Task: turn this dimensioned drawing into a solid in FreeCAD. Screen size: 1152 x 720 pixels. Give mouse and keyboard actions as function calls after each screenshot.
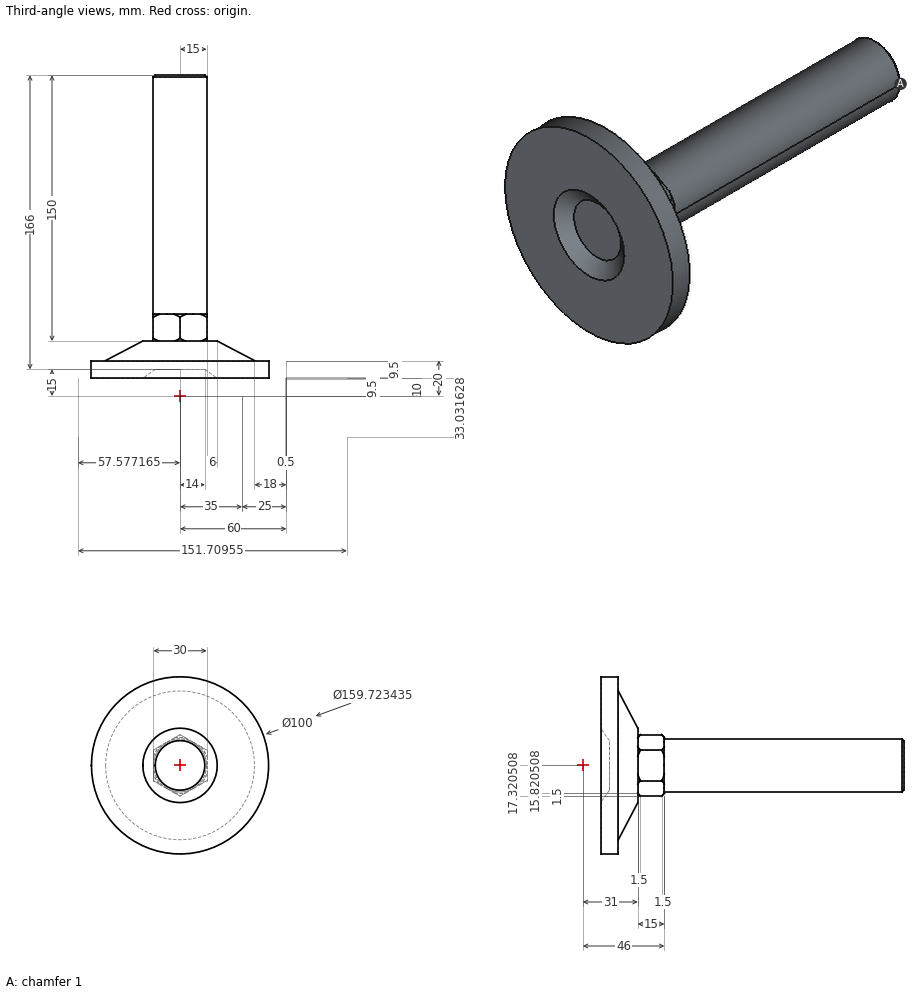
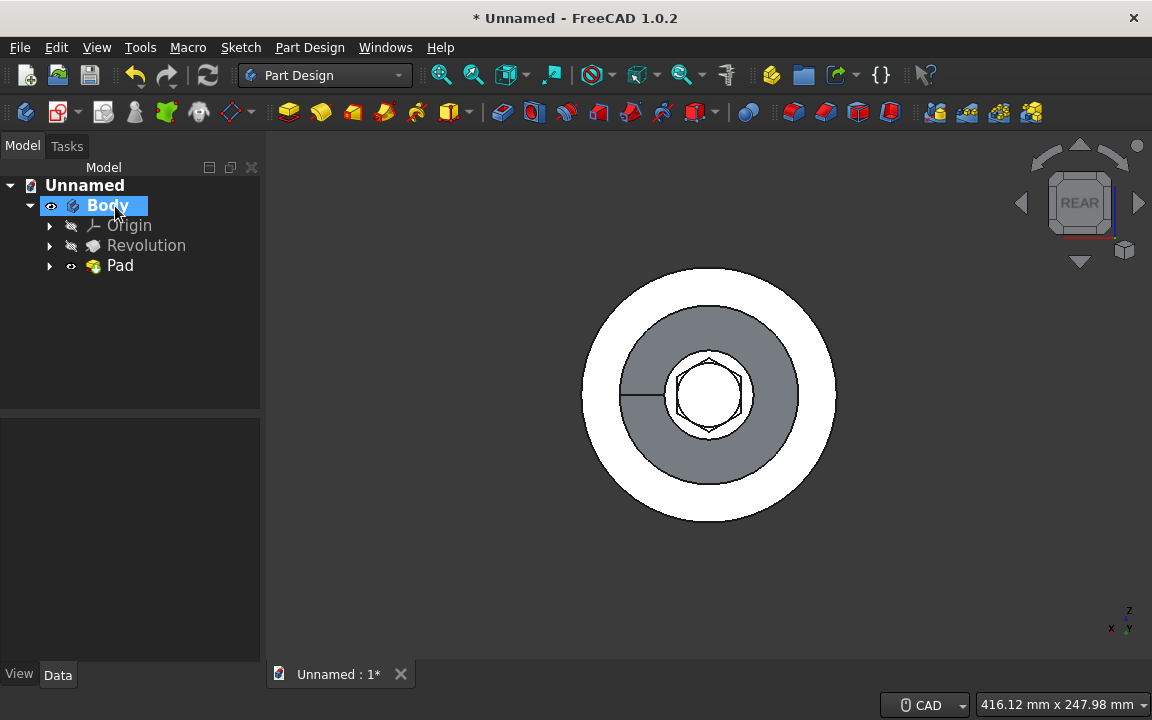
click(58, 112)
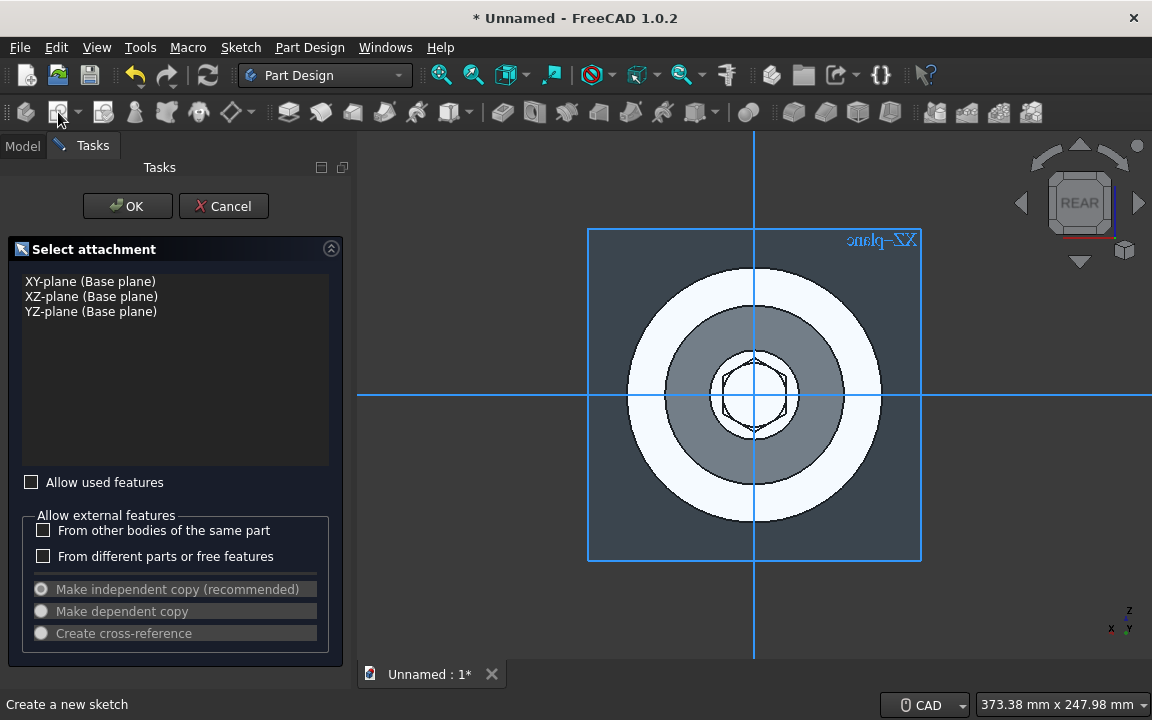
click(82, 312)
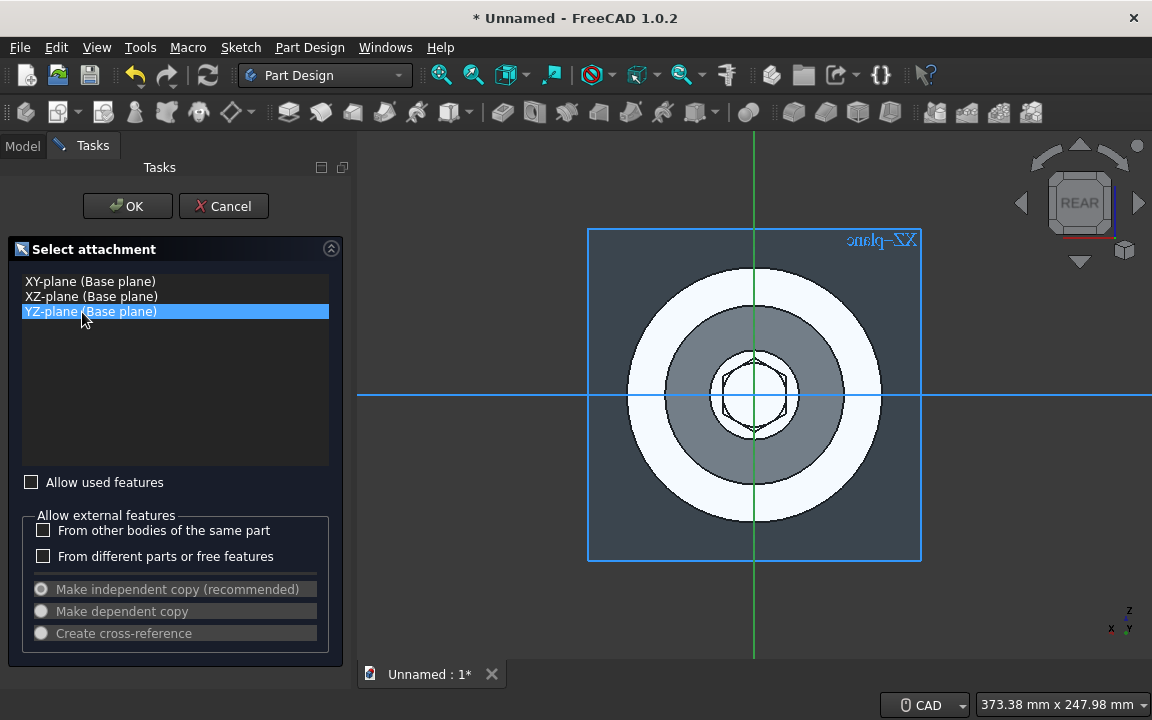
click(128, 206)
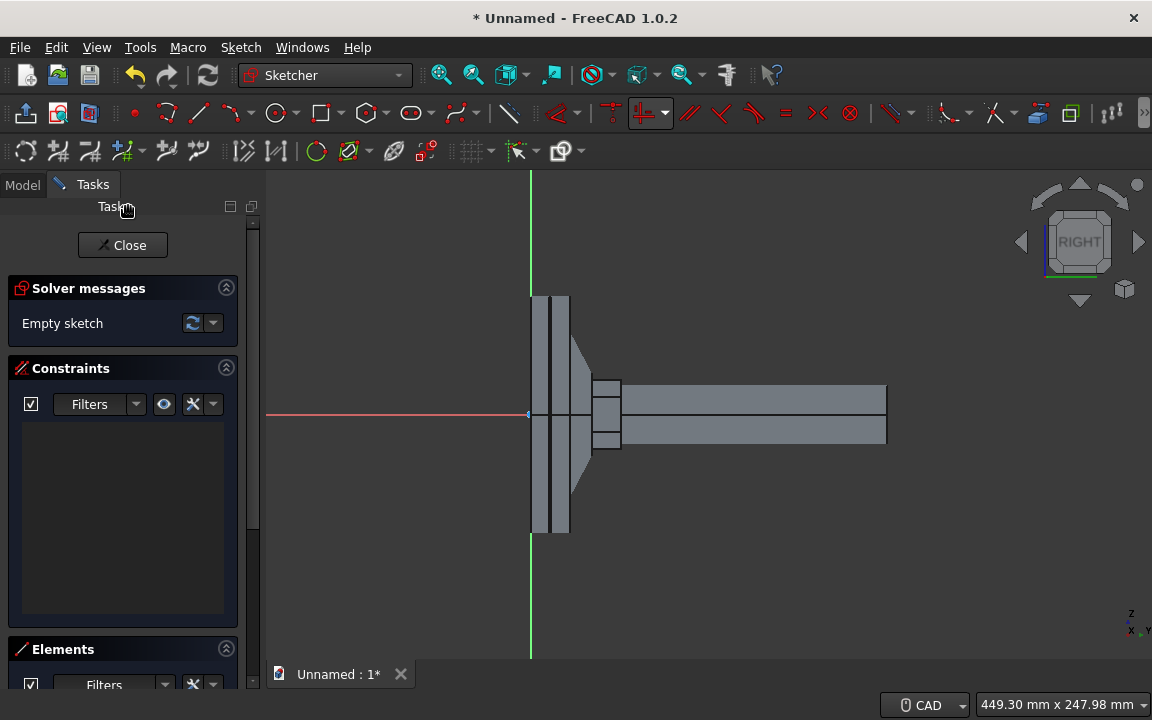
click(90, 114)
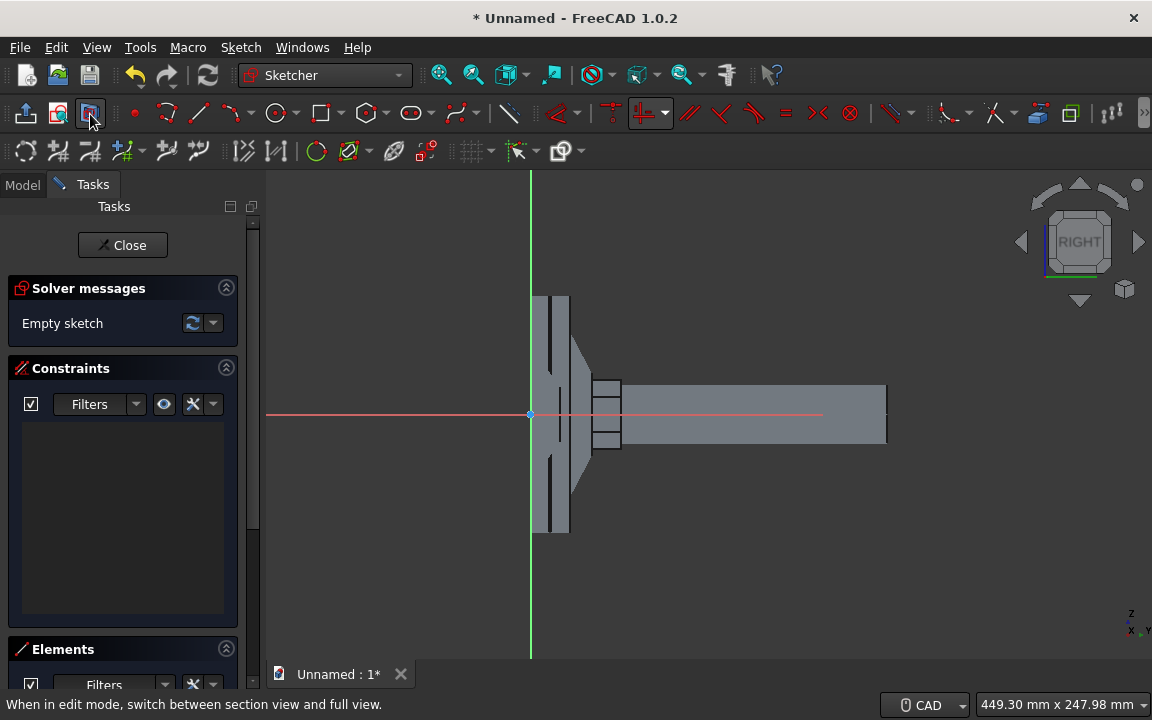
scroll(604, 449, up, 14)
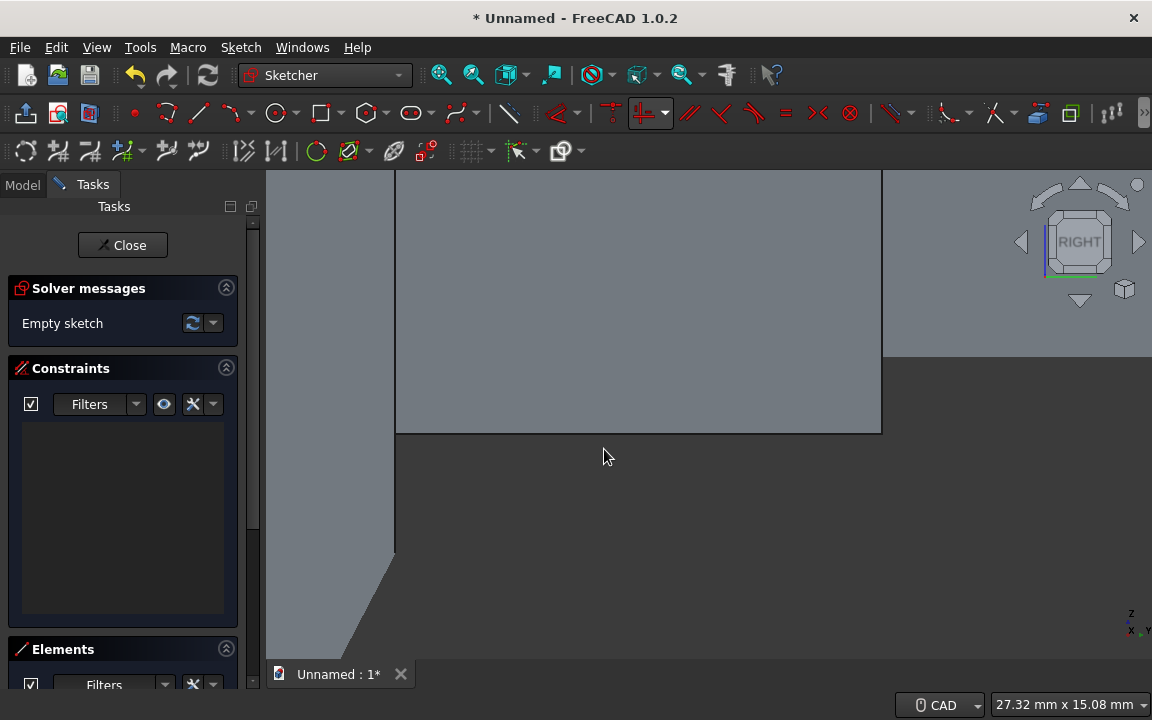
click(168, 114)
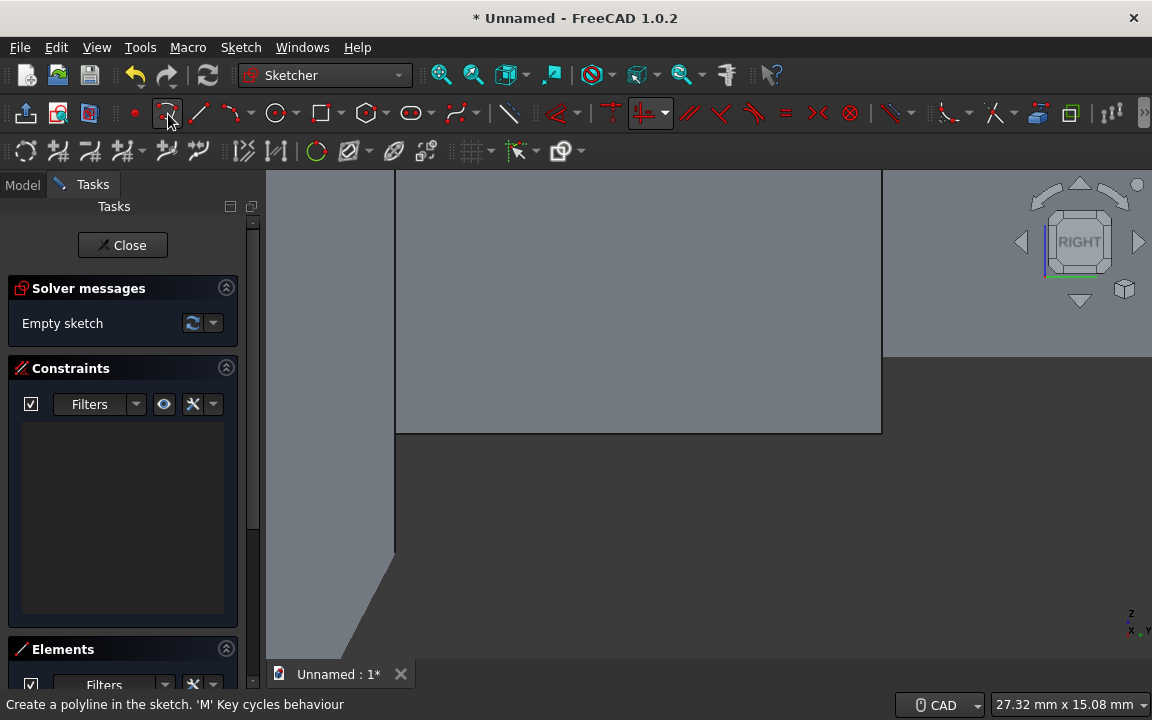
click(395, 386)
click(395, 434)
click(444, 434)
click(395, 387)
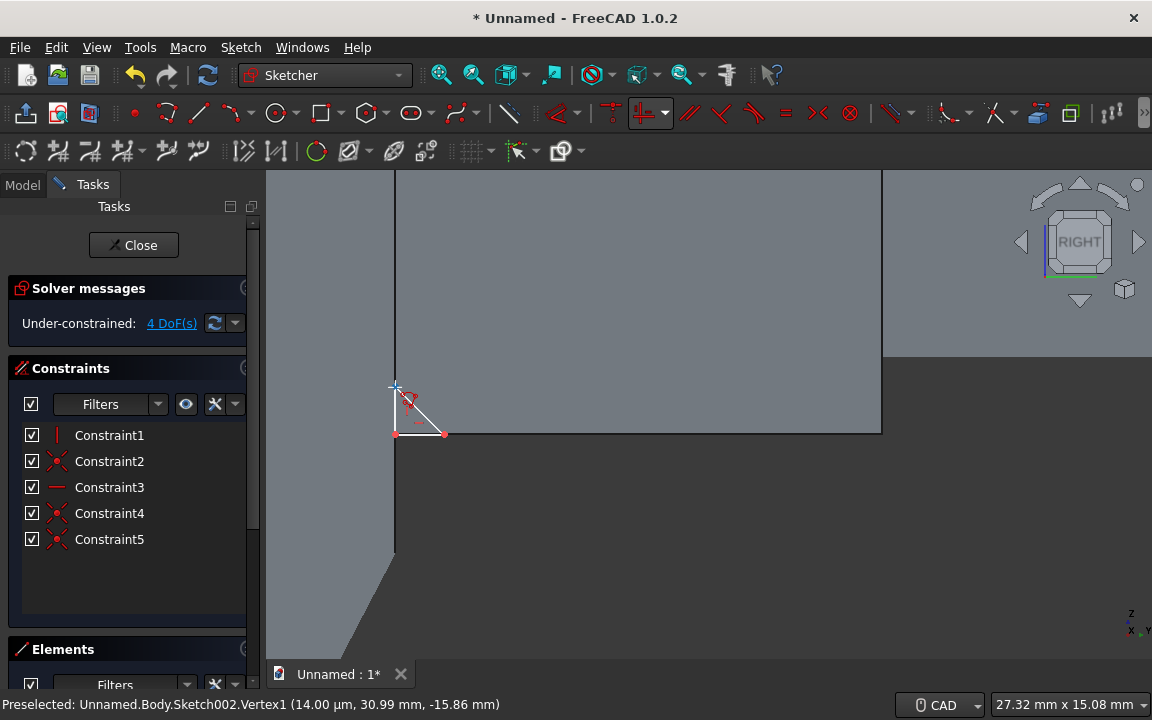
click(833, 434)
click(882, 434)
click(882, 386)
click(833, 435)
key(Escape)
key(Escape)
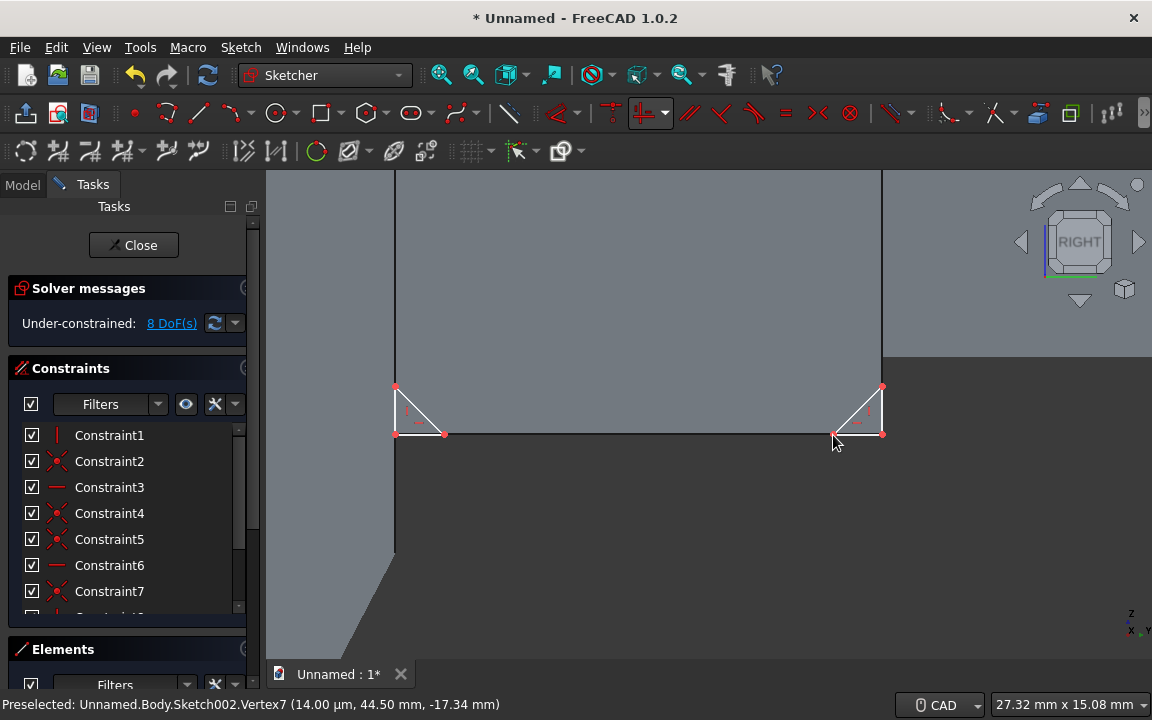
click(556, 114)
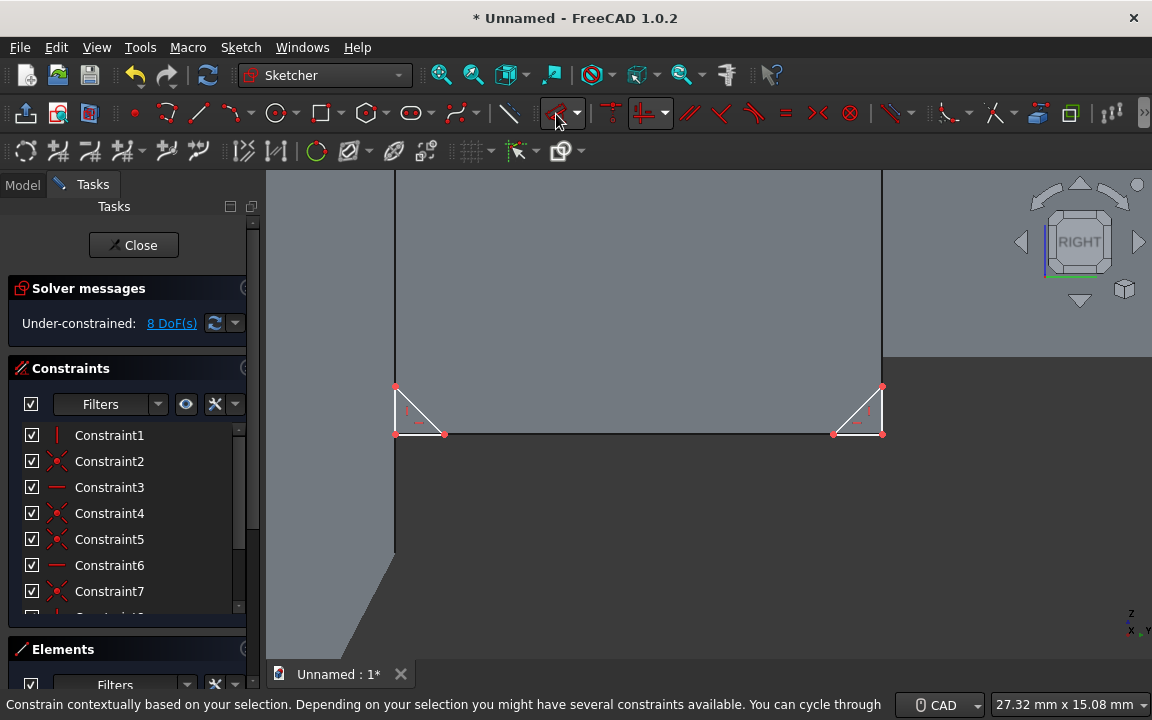
scroll(395, 401, up, 2)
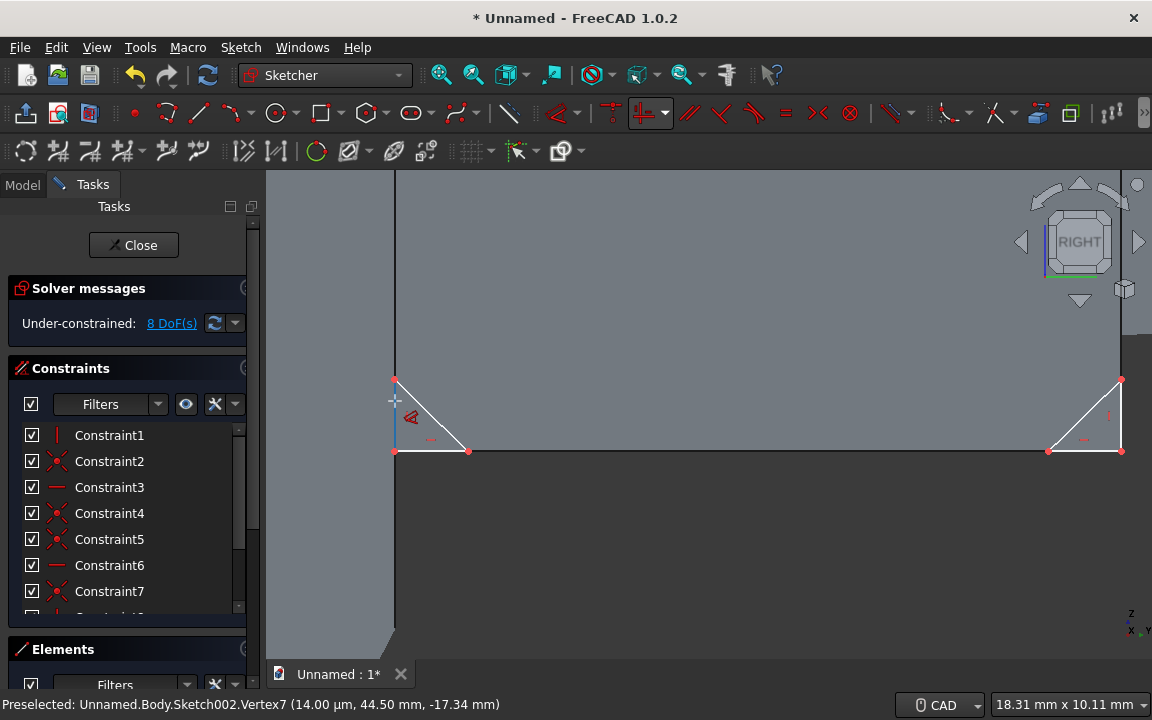
click(395, 401)
click(361, 416)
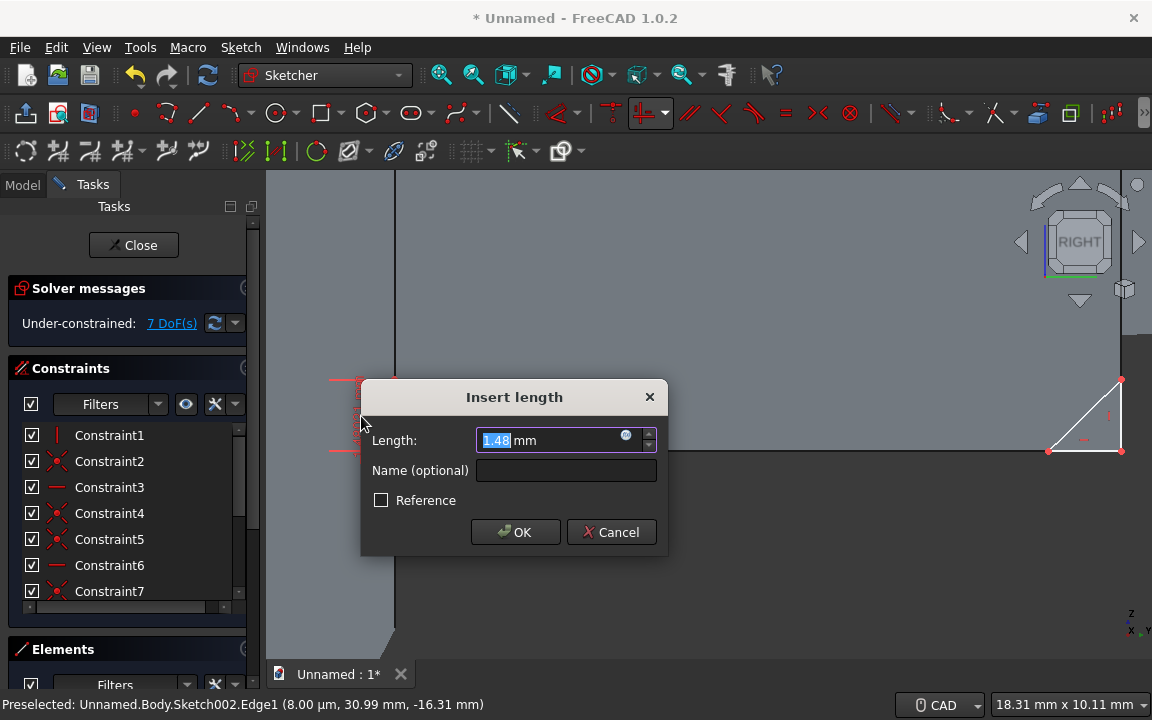
text(1.5)
key(Return)